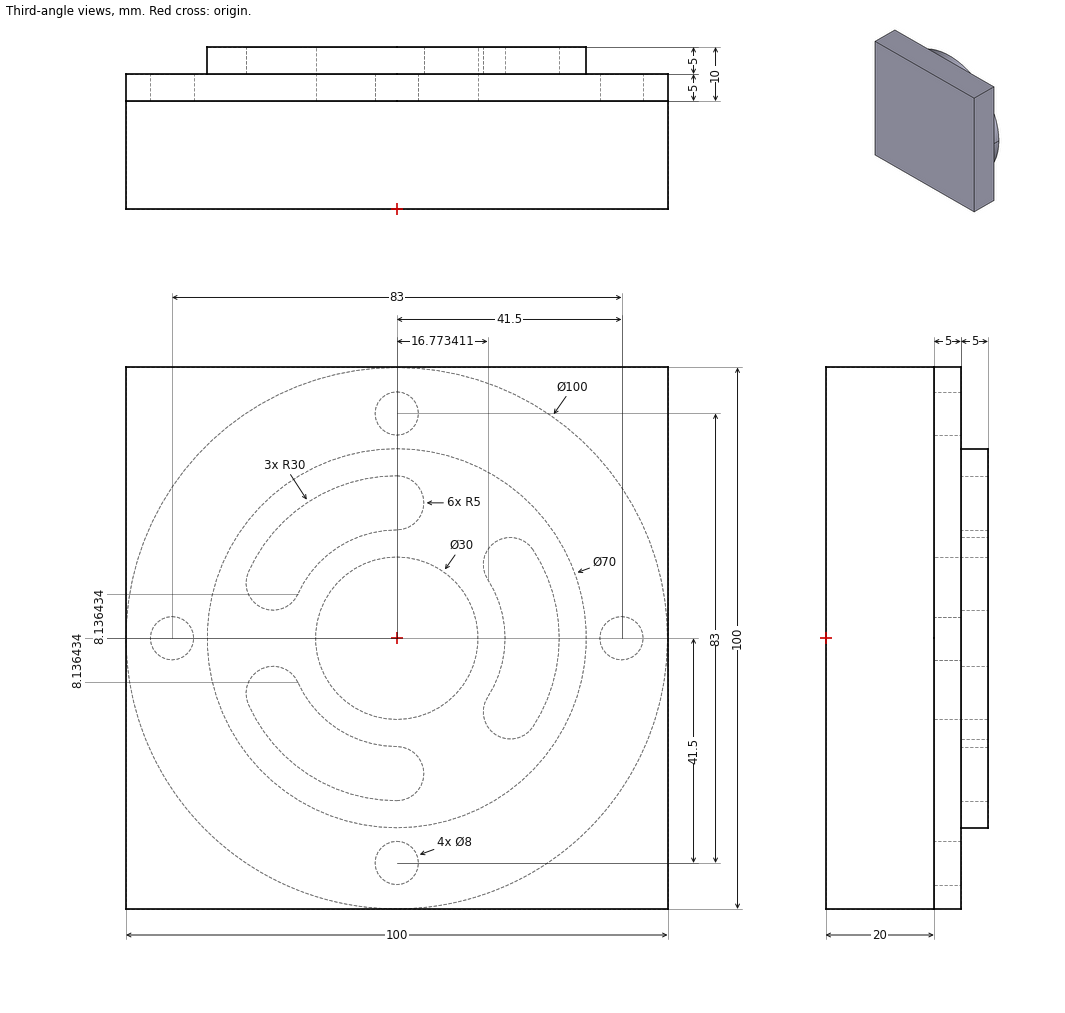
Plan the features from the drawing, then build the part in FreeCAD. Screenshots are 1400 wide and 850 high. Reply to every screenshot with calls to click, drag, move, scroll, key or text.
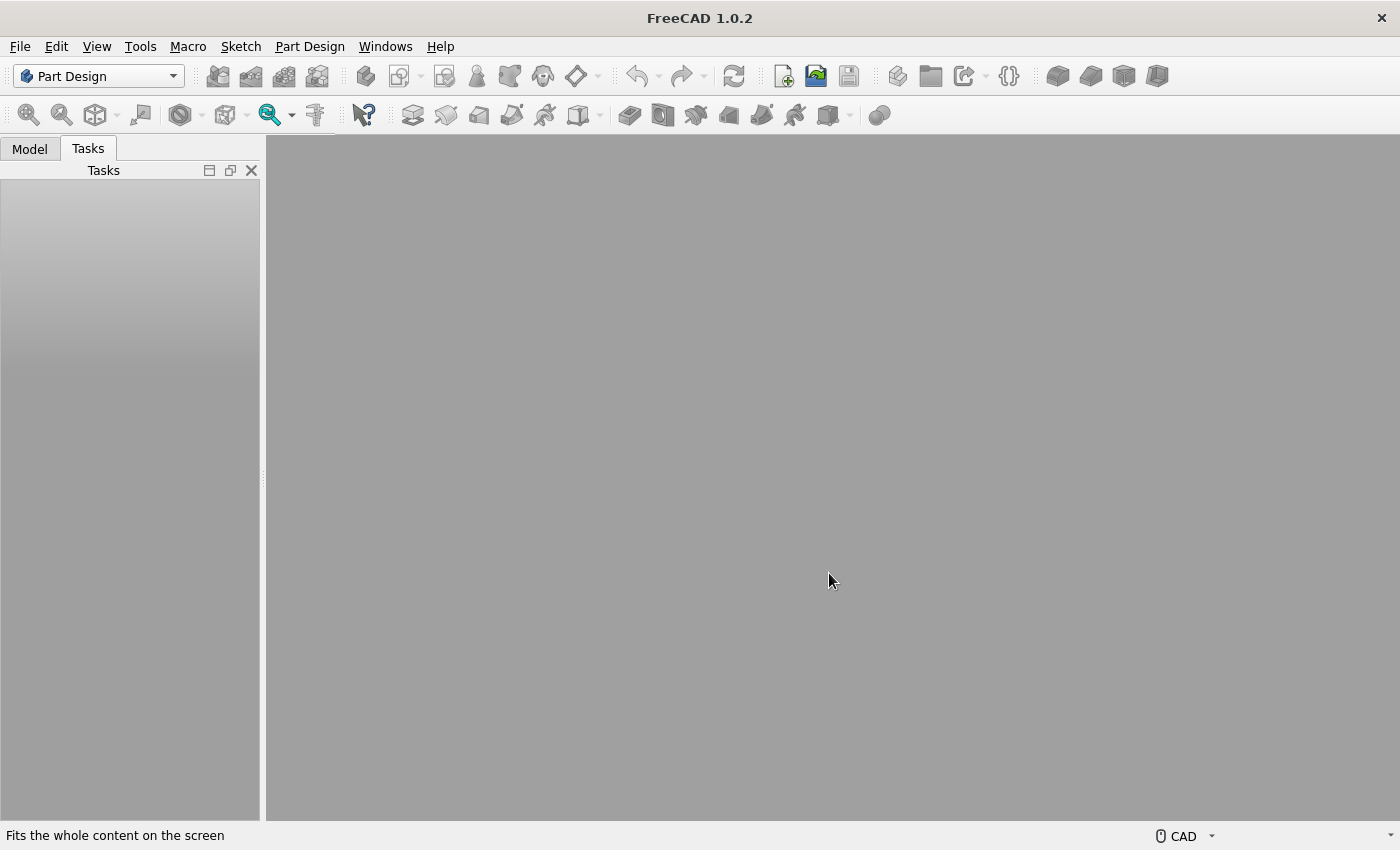
click(783, 76)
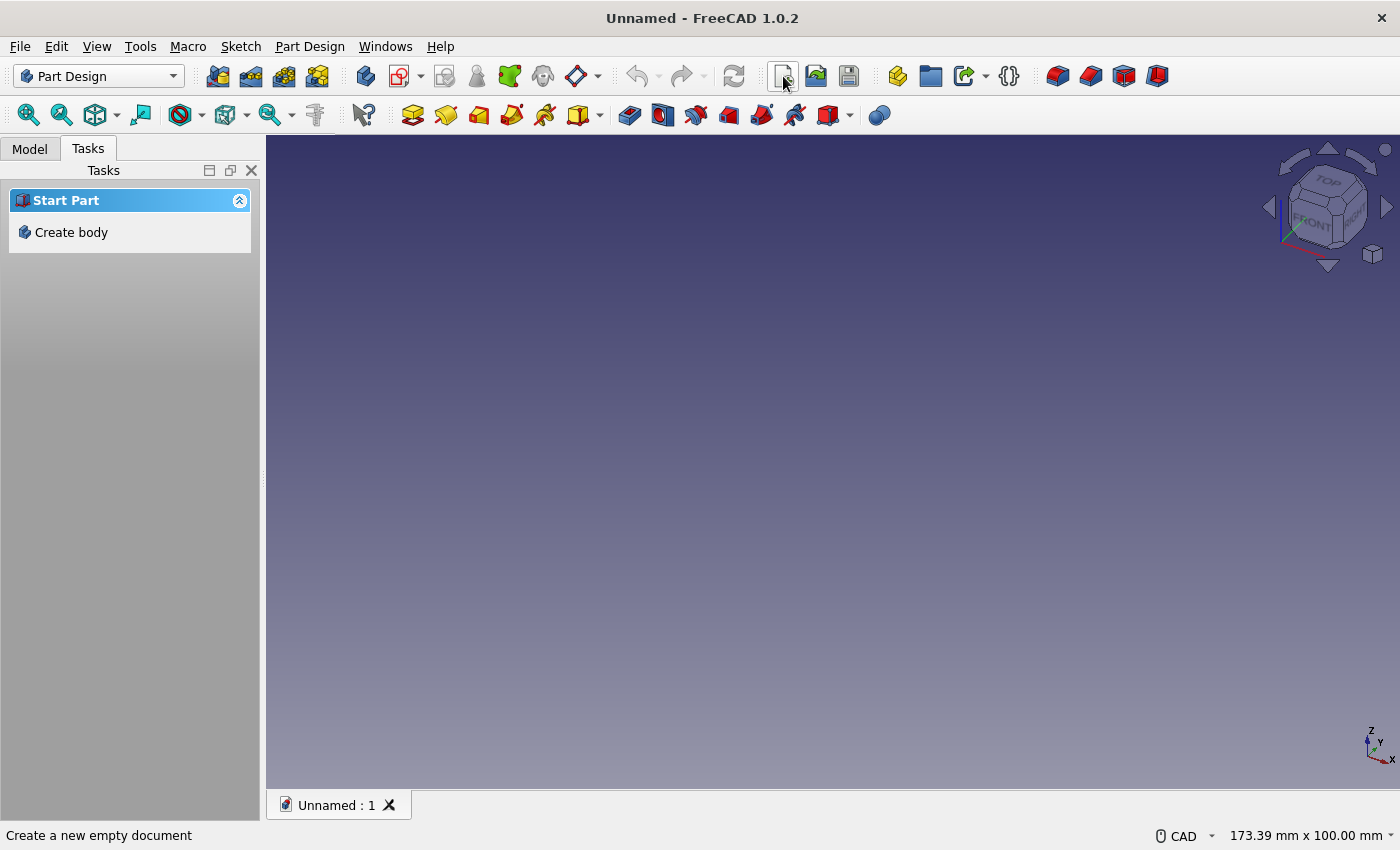
click(398, 76)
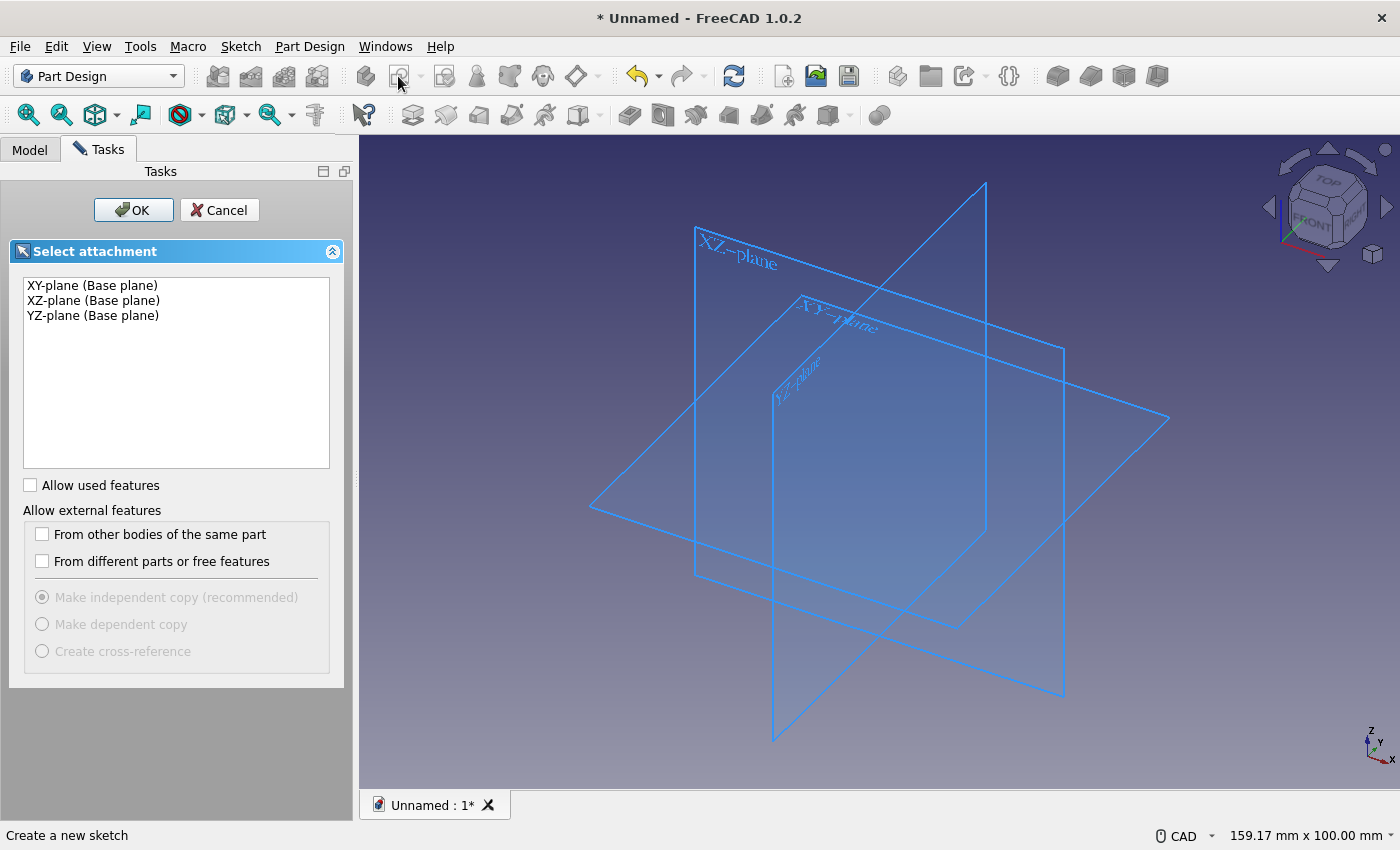
click(84, 300)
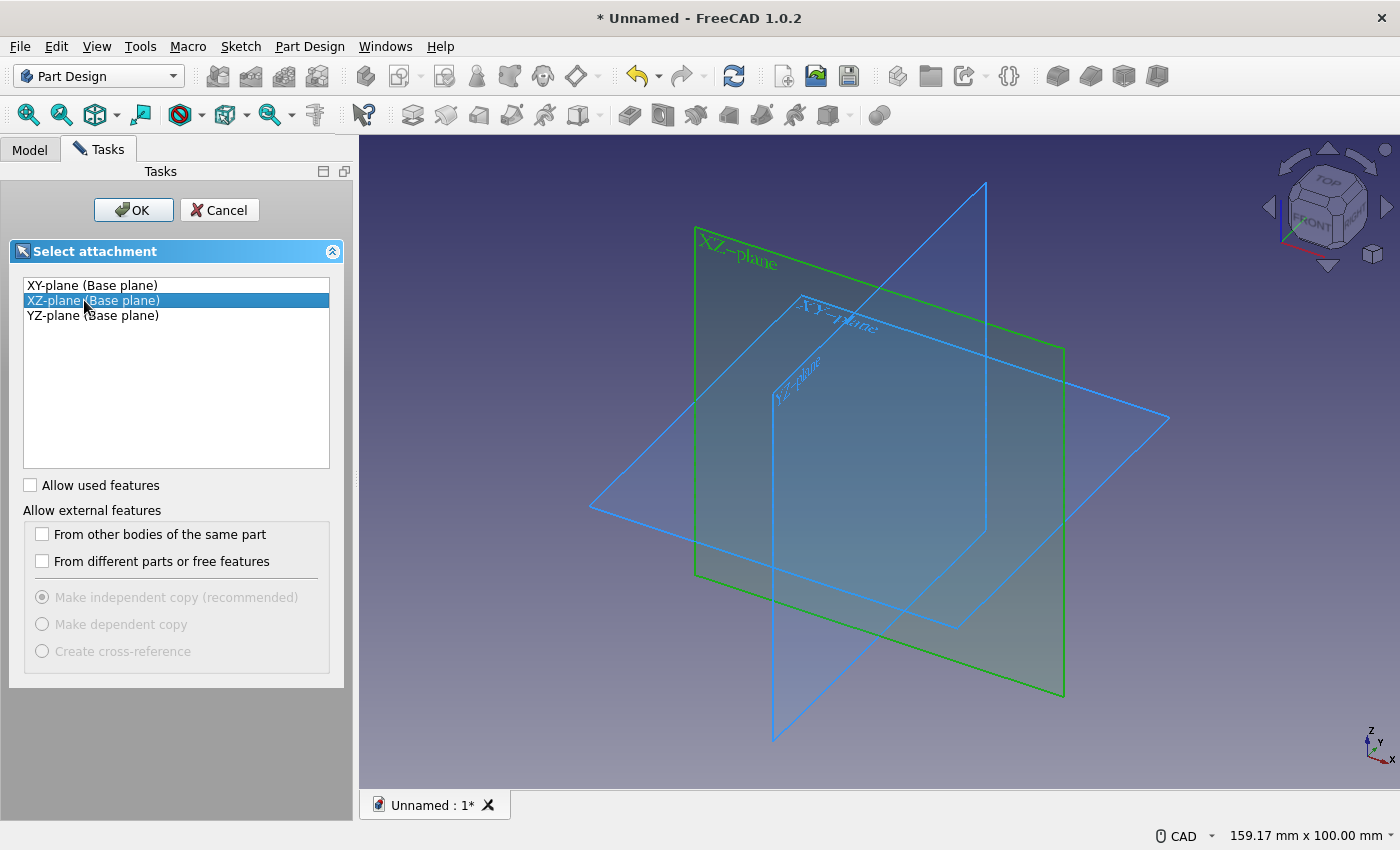
click(134, 210)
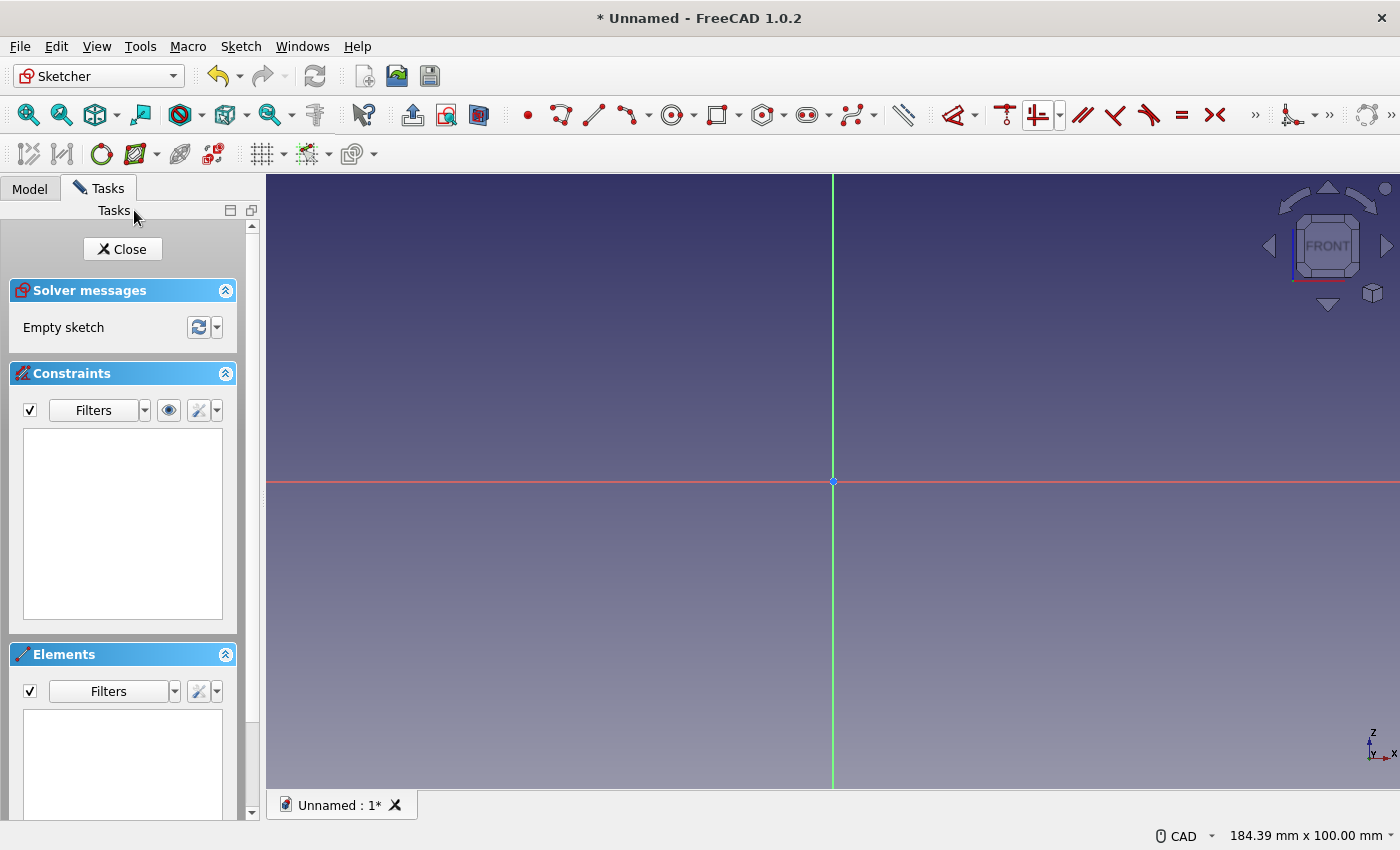
scroll(625, 481, down, 2)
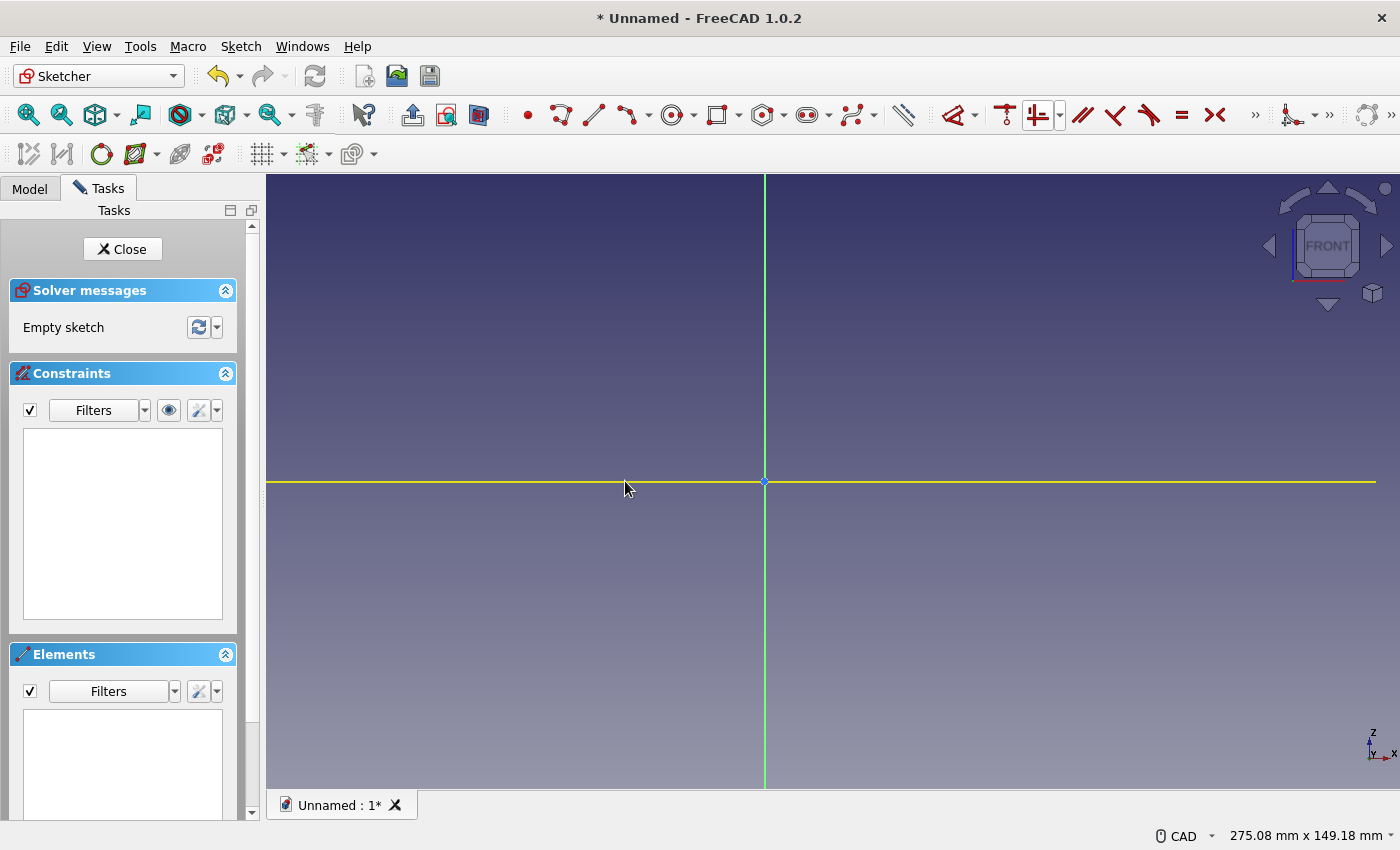
click(738, 116)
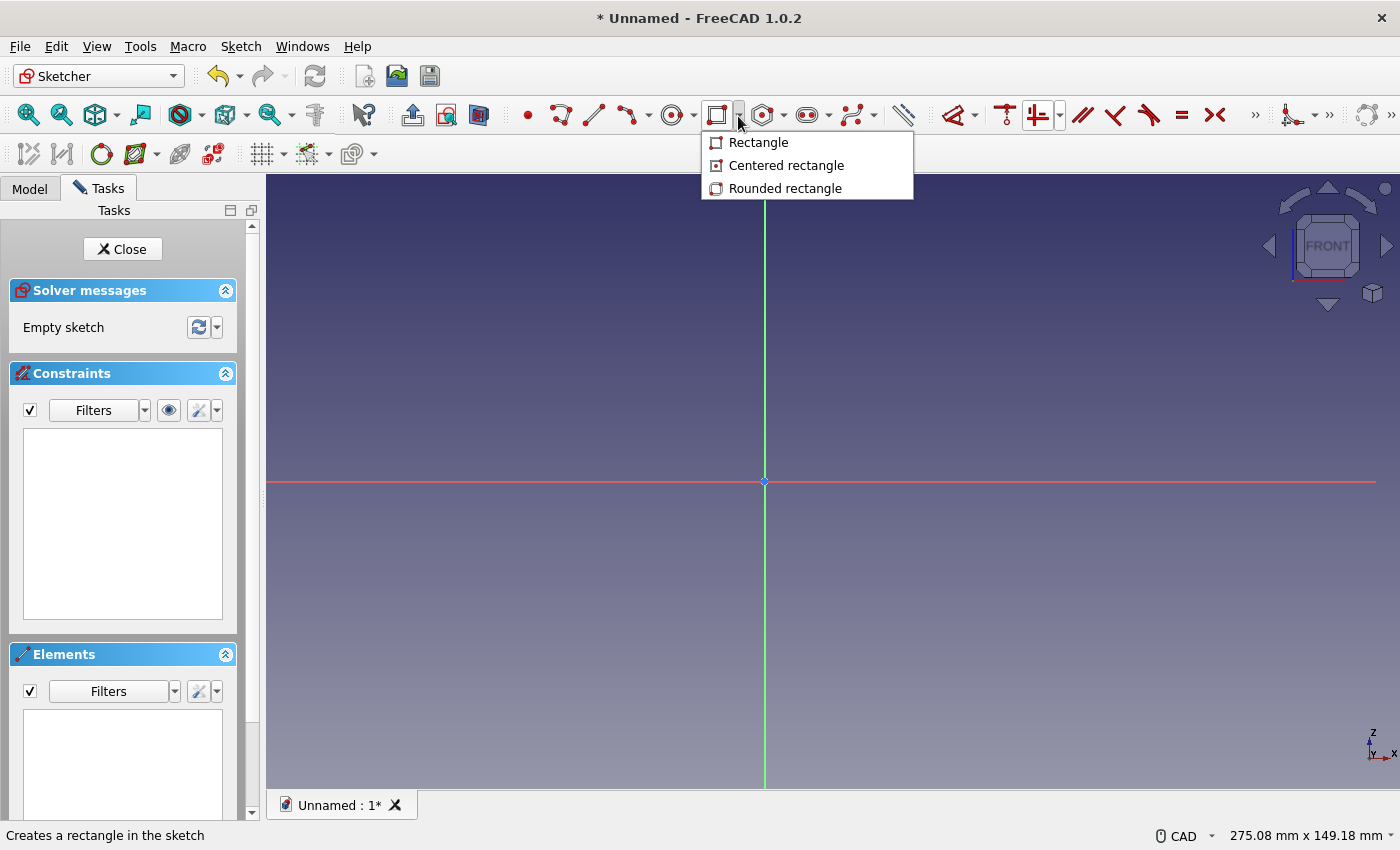
click(808, 166)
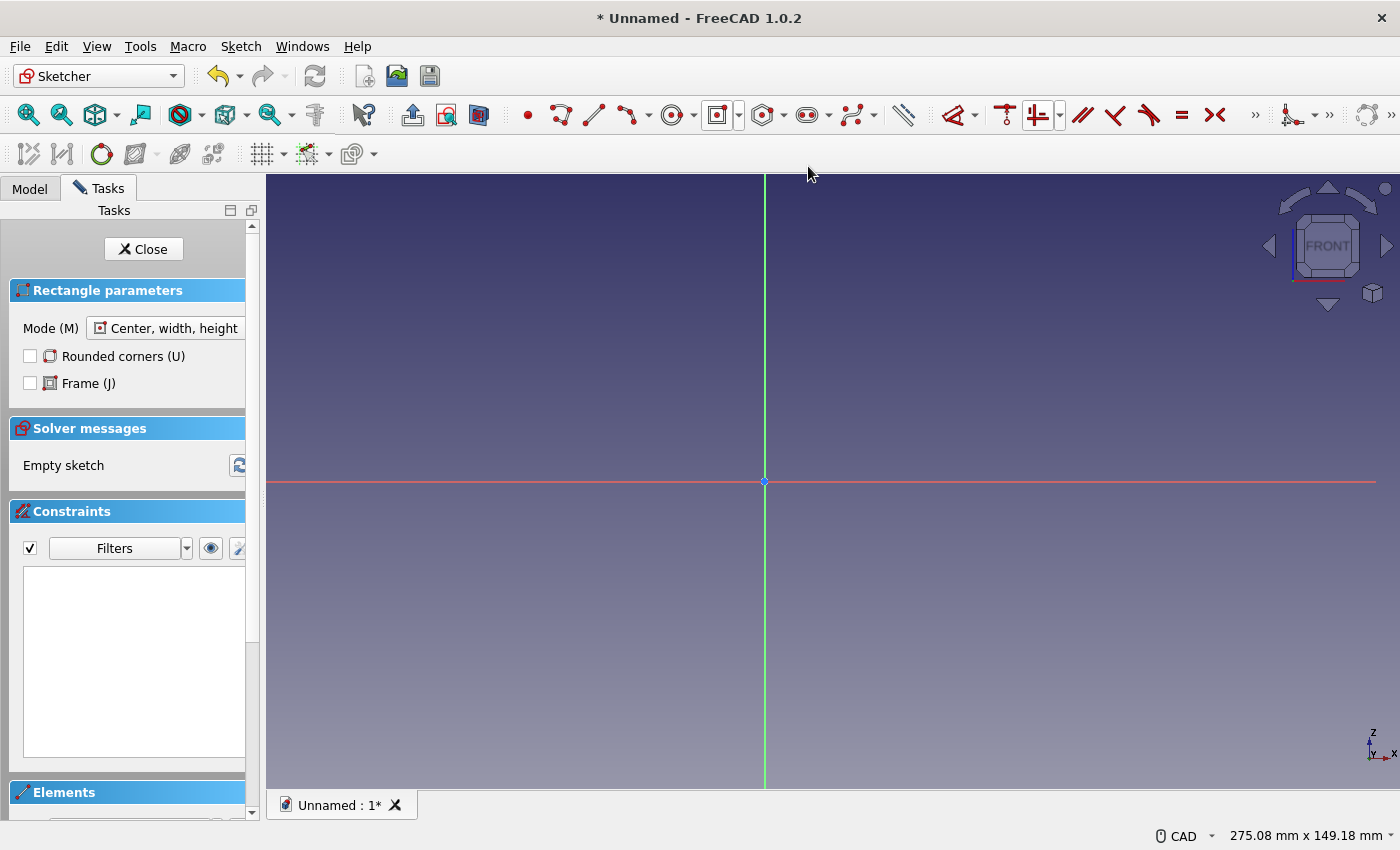
click(765, 482)
move(971, 275)